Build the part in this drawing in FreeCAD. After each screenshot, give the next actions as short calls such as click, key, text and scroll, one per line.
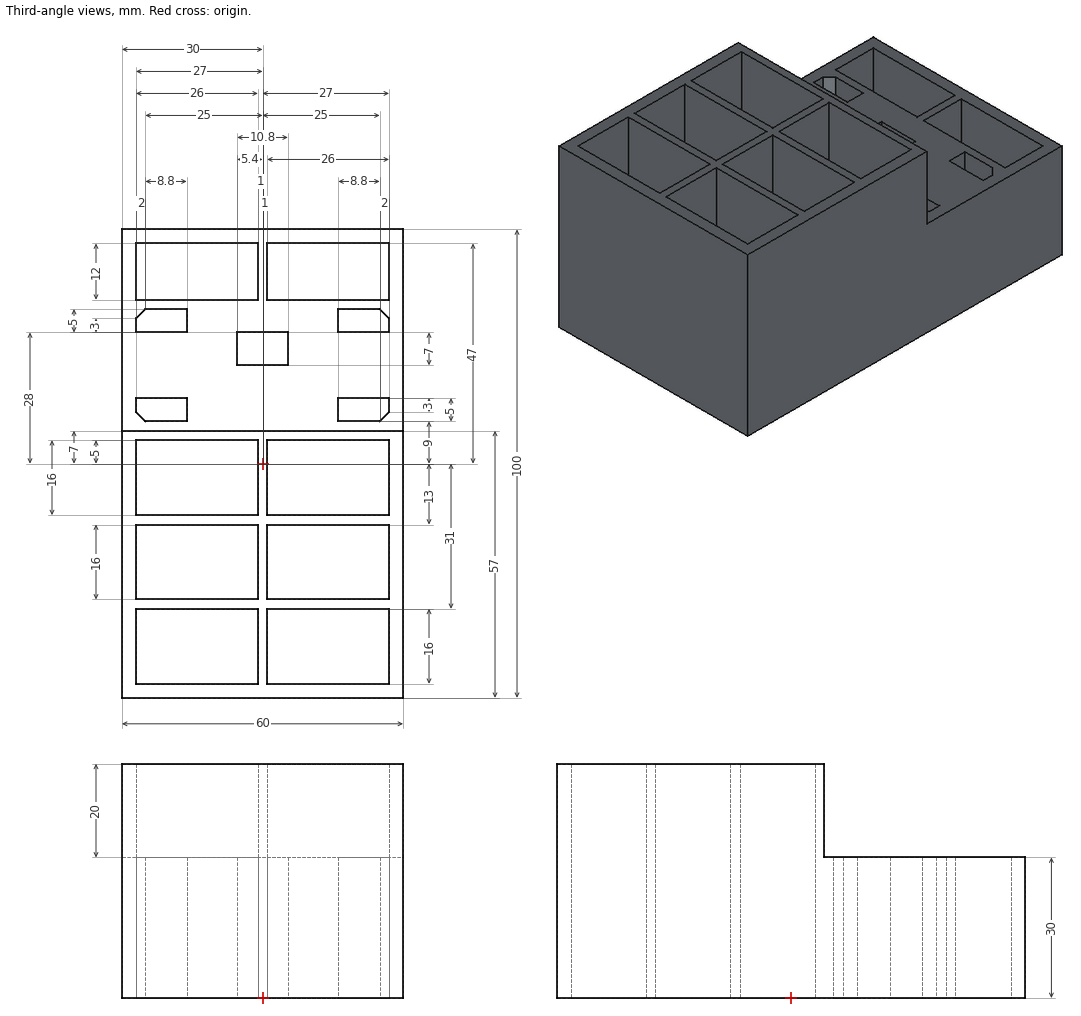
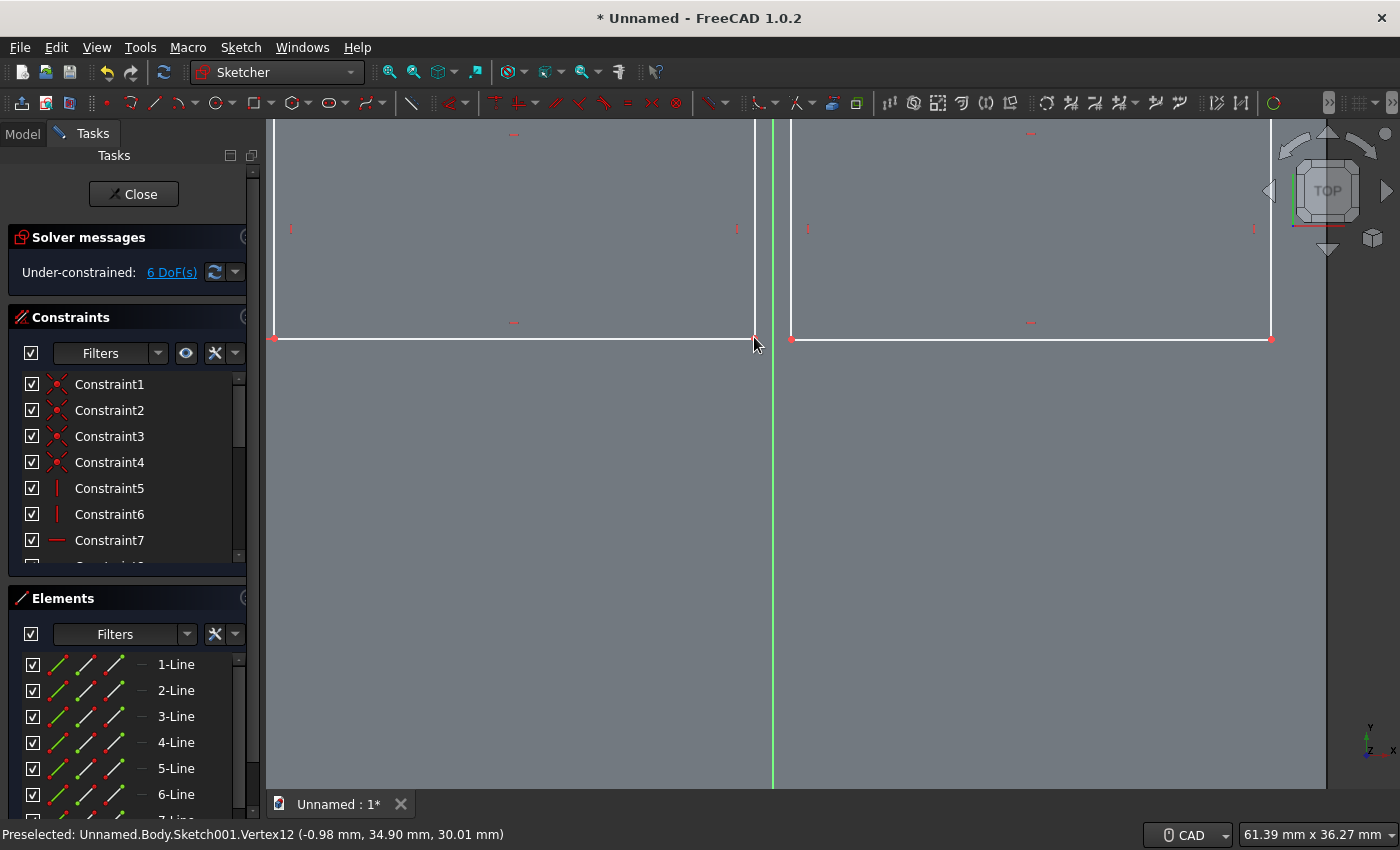
click(450, 104)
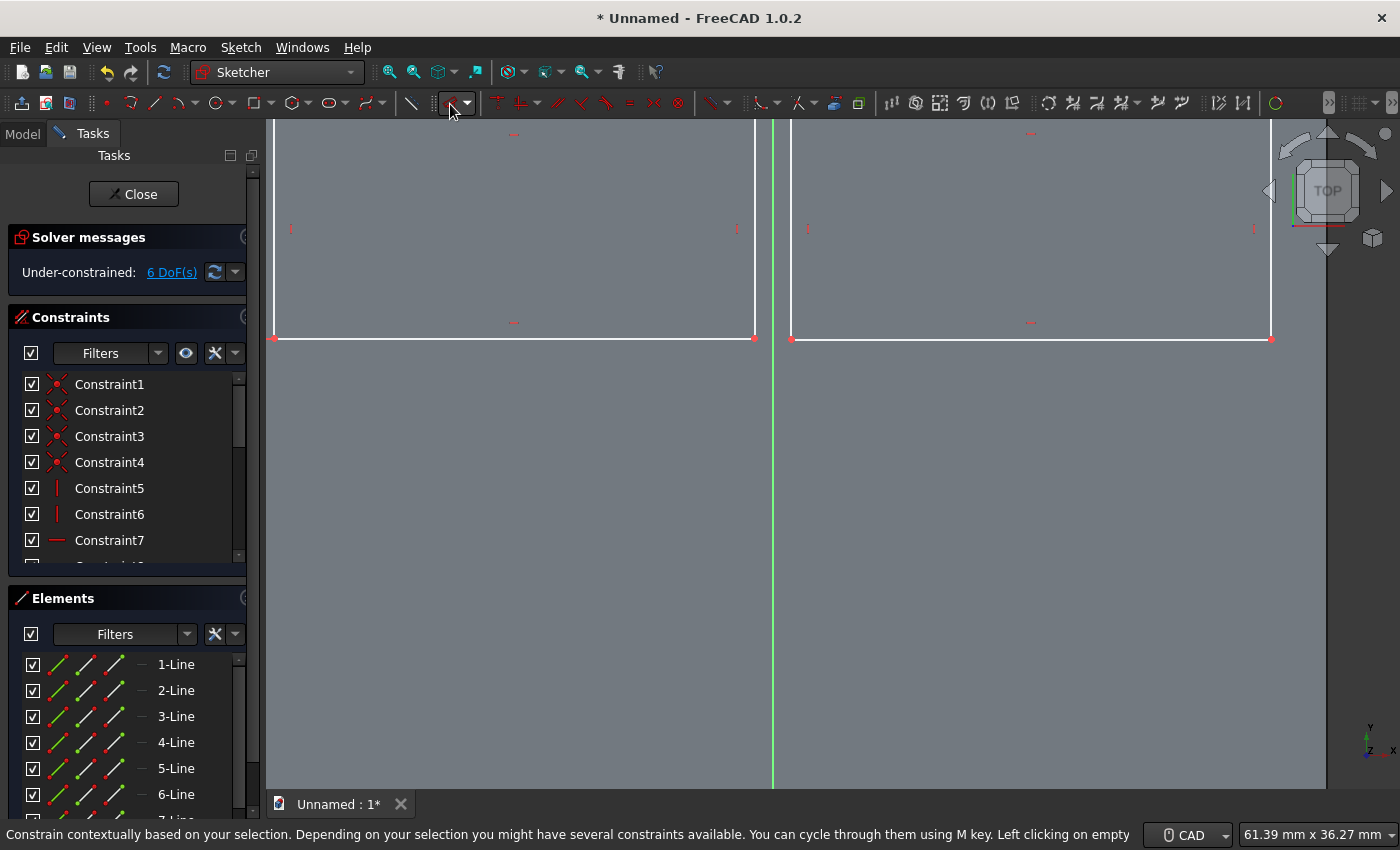
click(791, 183)
click(825, 243)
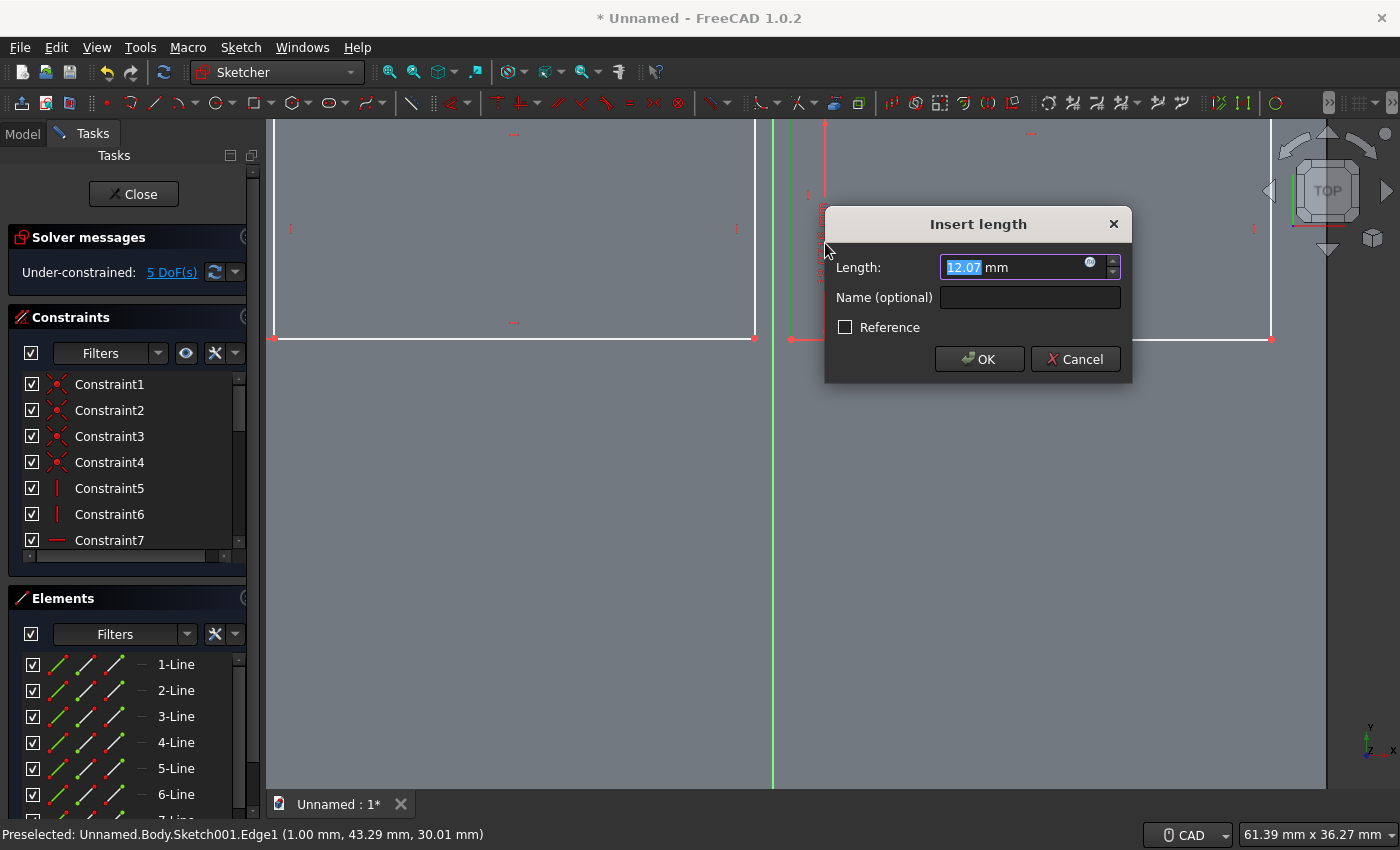
text(12)
key(Return)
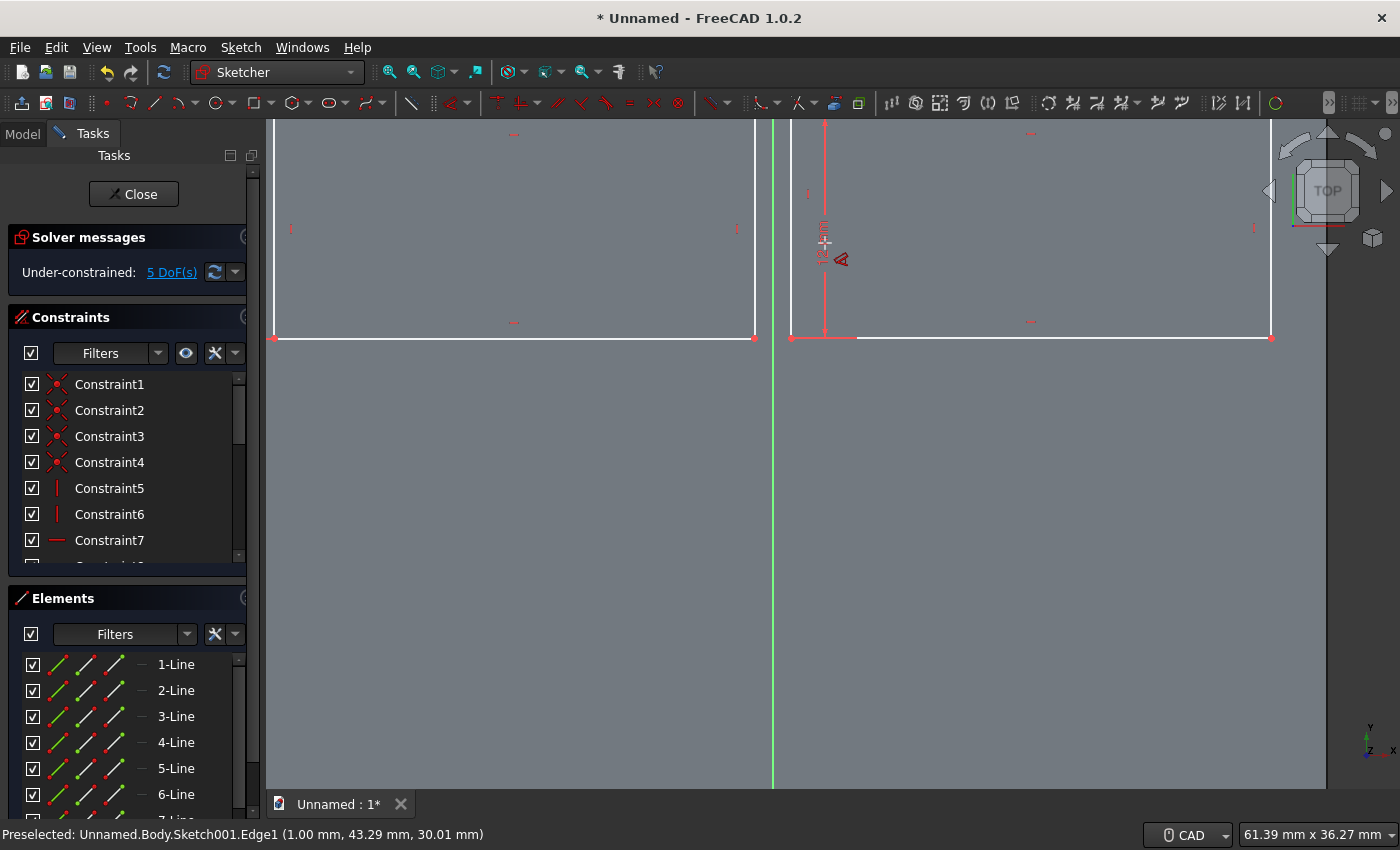
click(935, 338)
click(1013, 304)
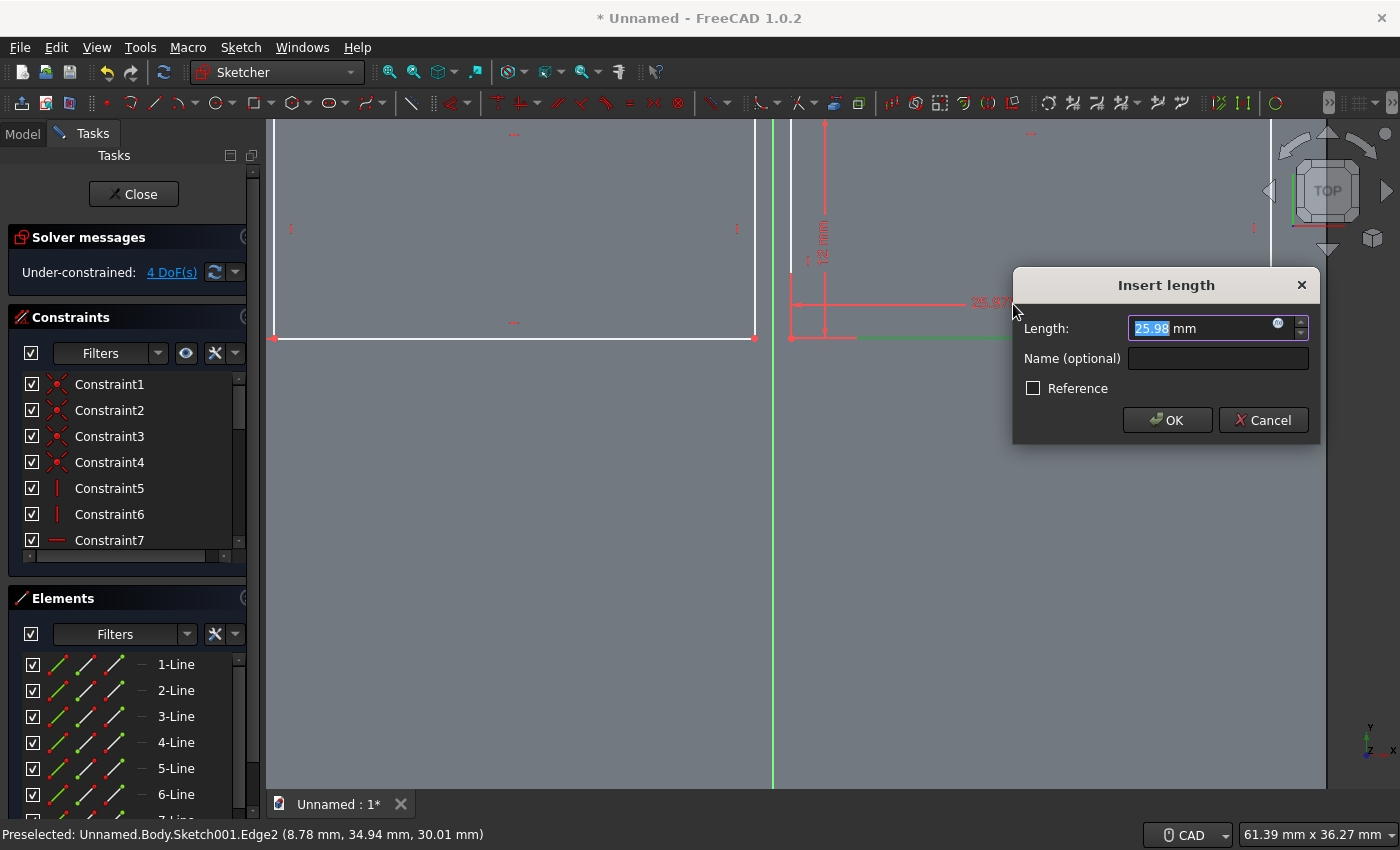
text(26)
key(Return)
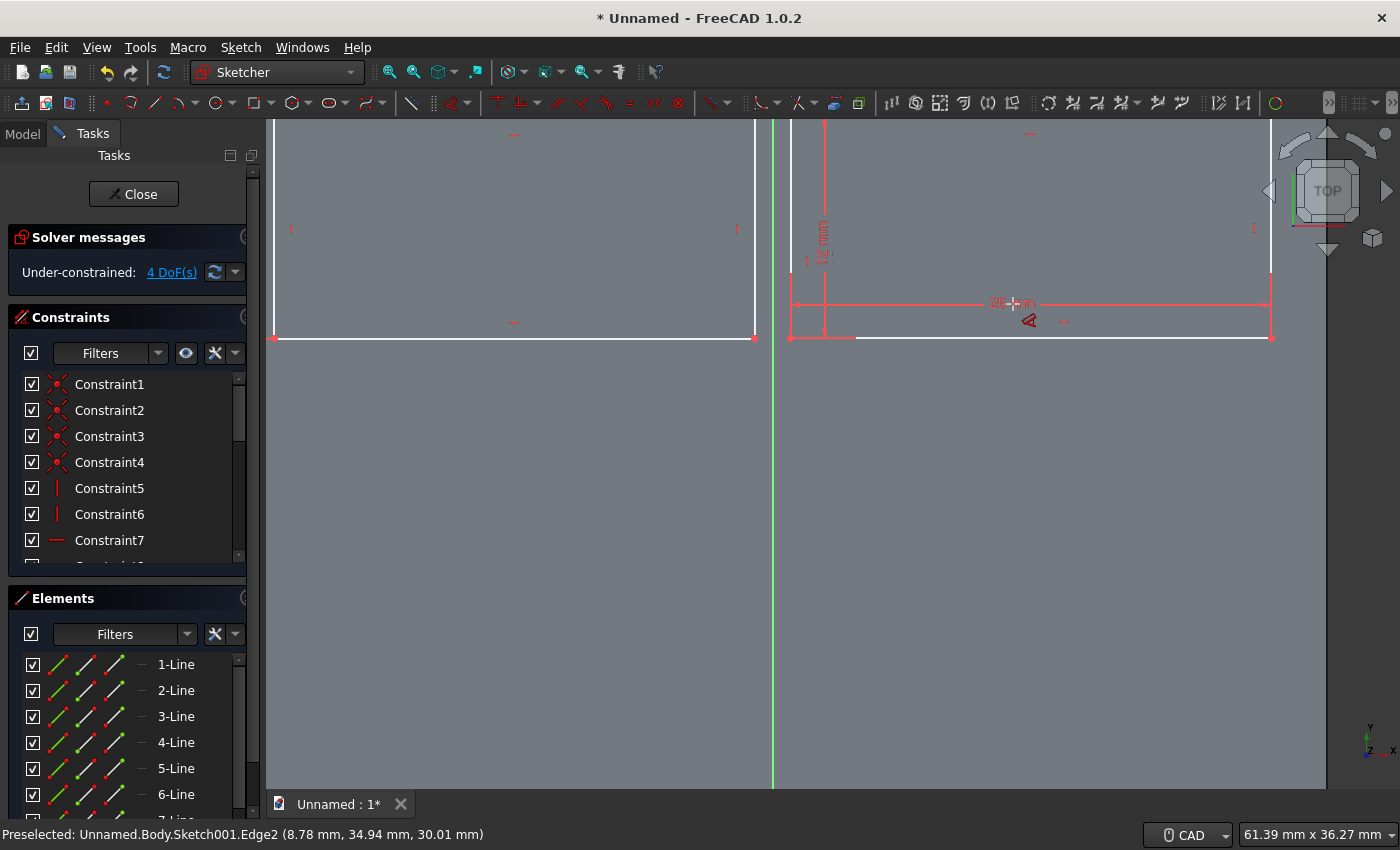
scroll(754, 338, down, 3)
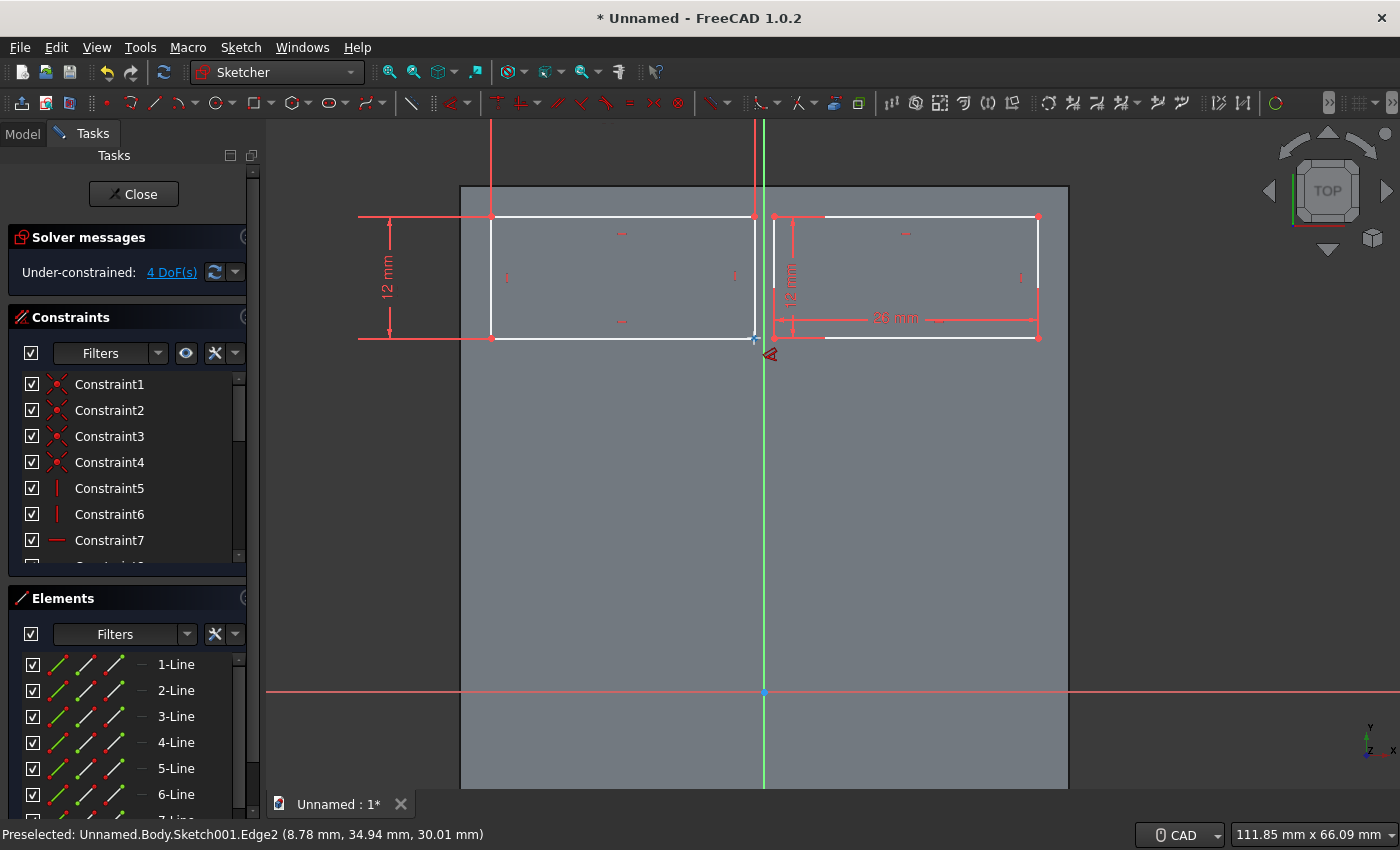
scroll(774, 217, up, 7)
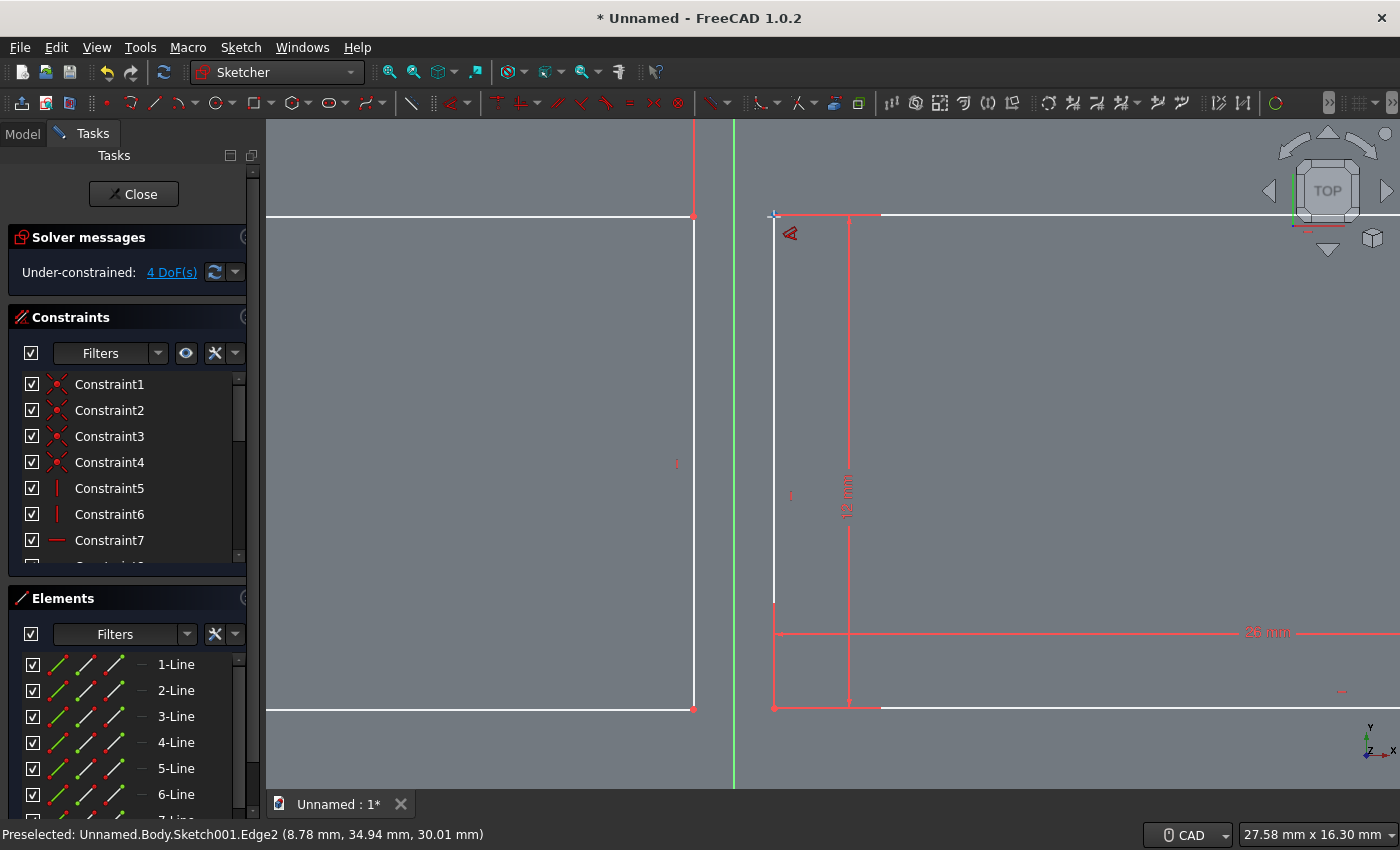
click(774, 215)
click(754, 181)